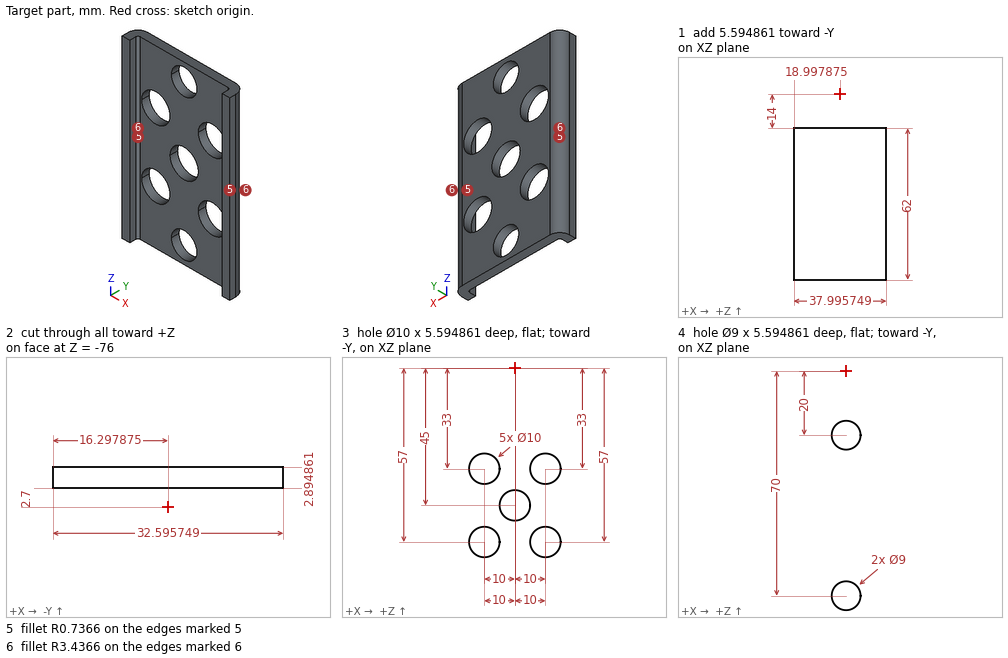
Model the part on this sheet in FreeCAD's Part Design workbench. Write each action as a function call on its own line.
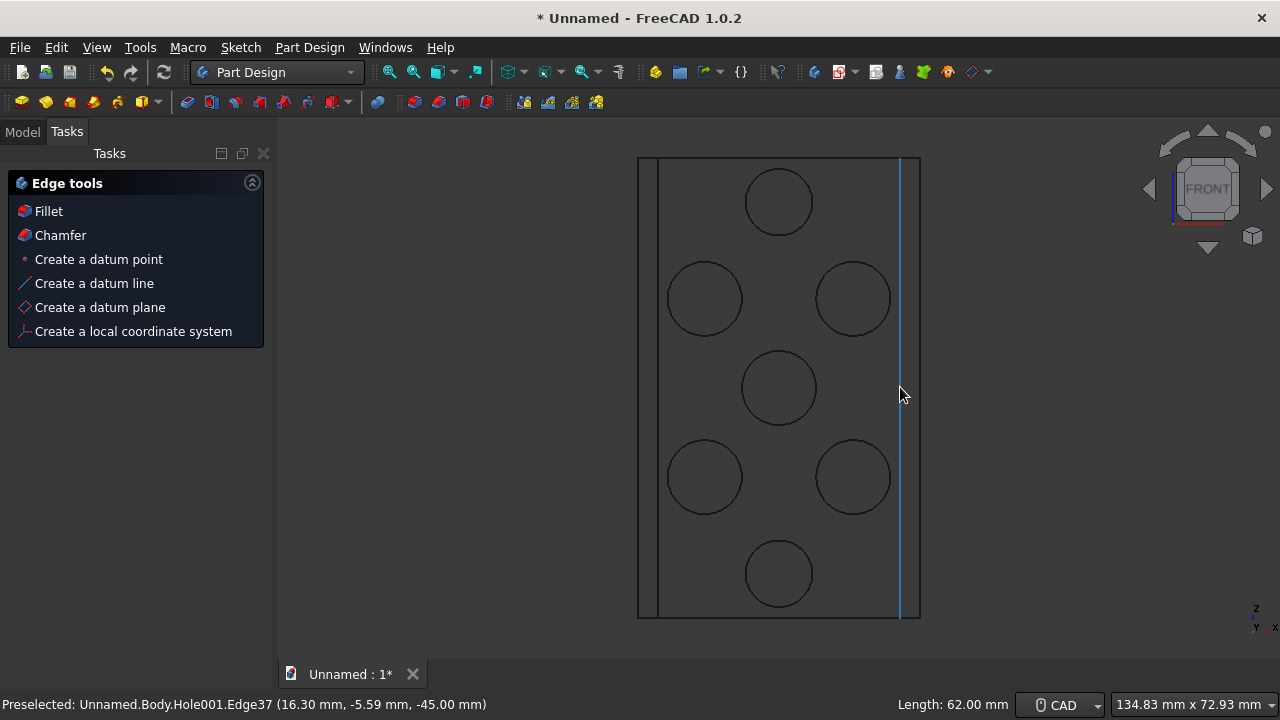
key(3)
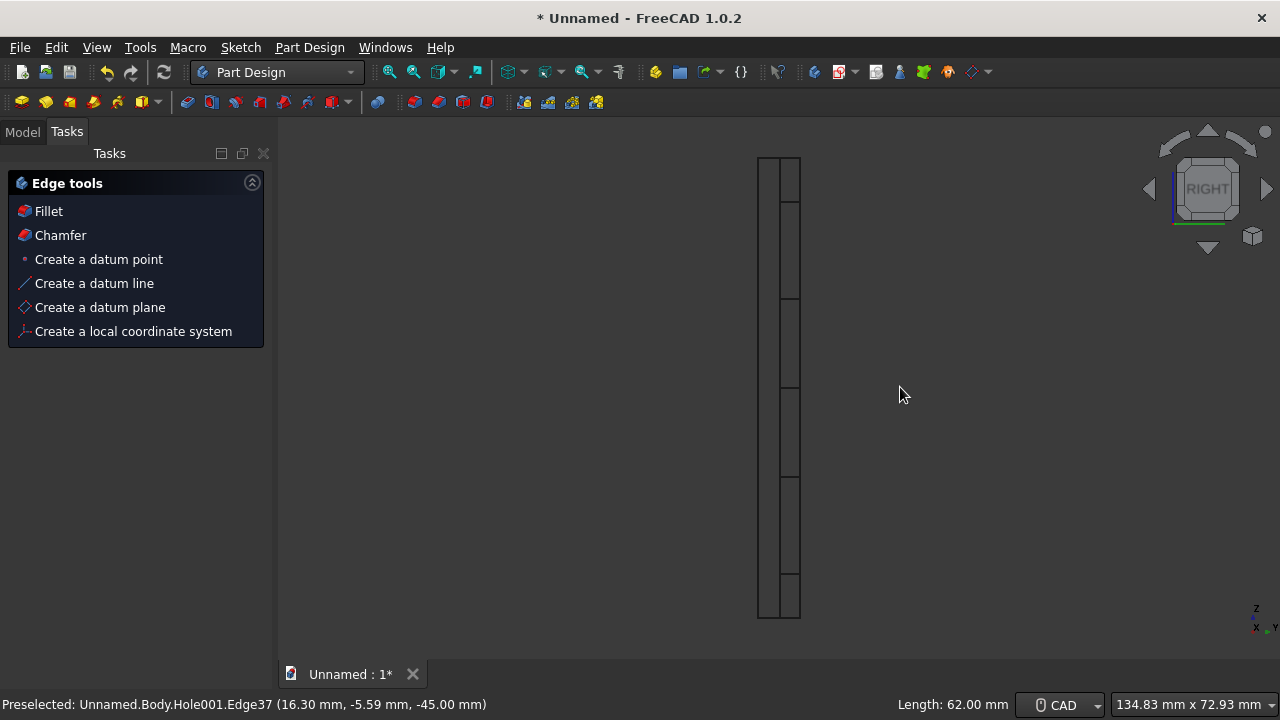
click(780, 387, ctrl)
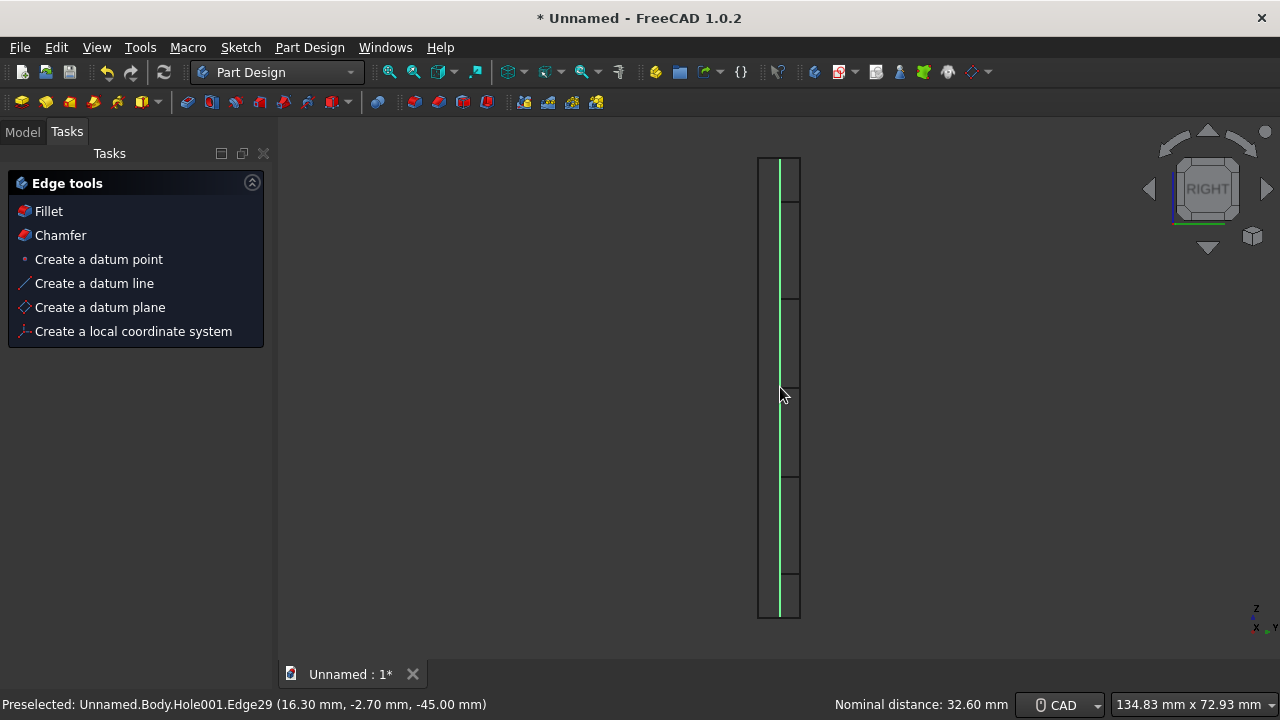
key(v)
key(1)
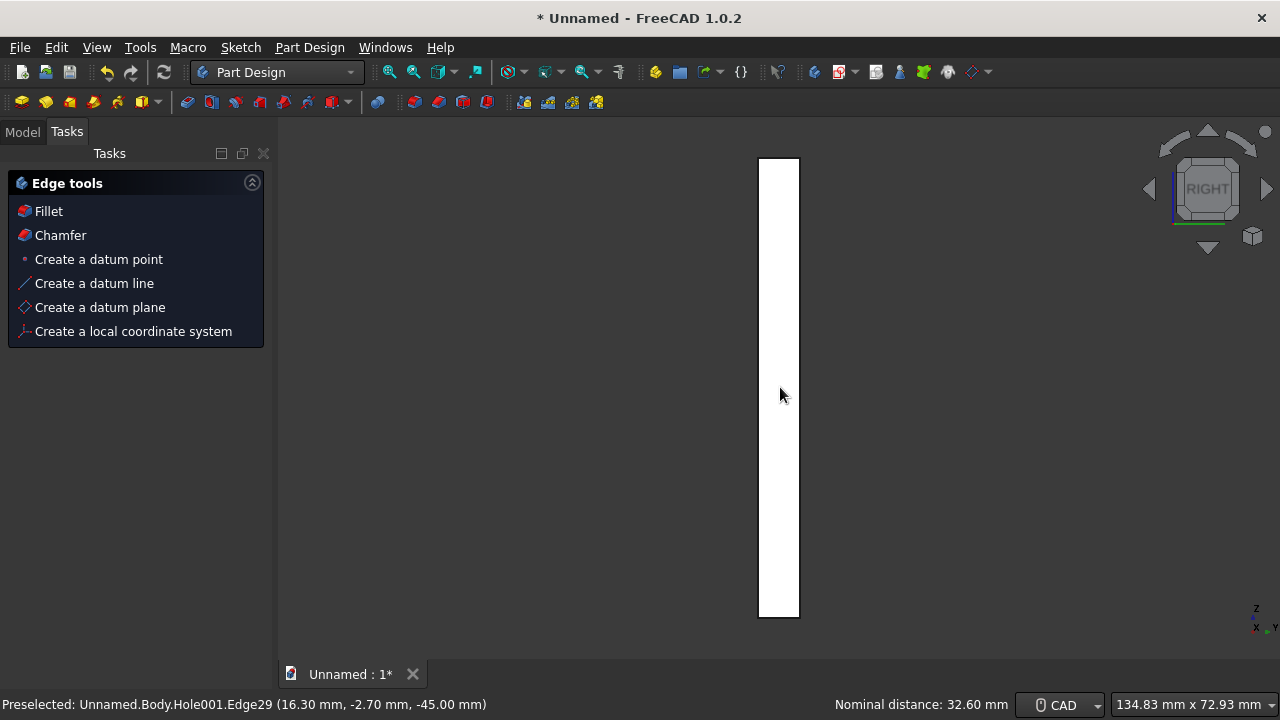
click(416, 102)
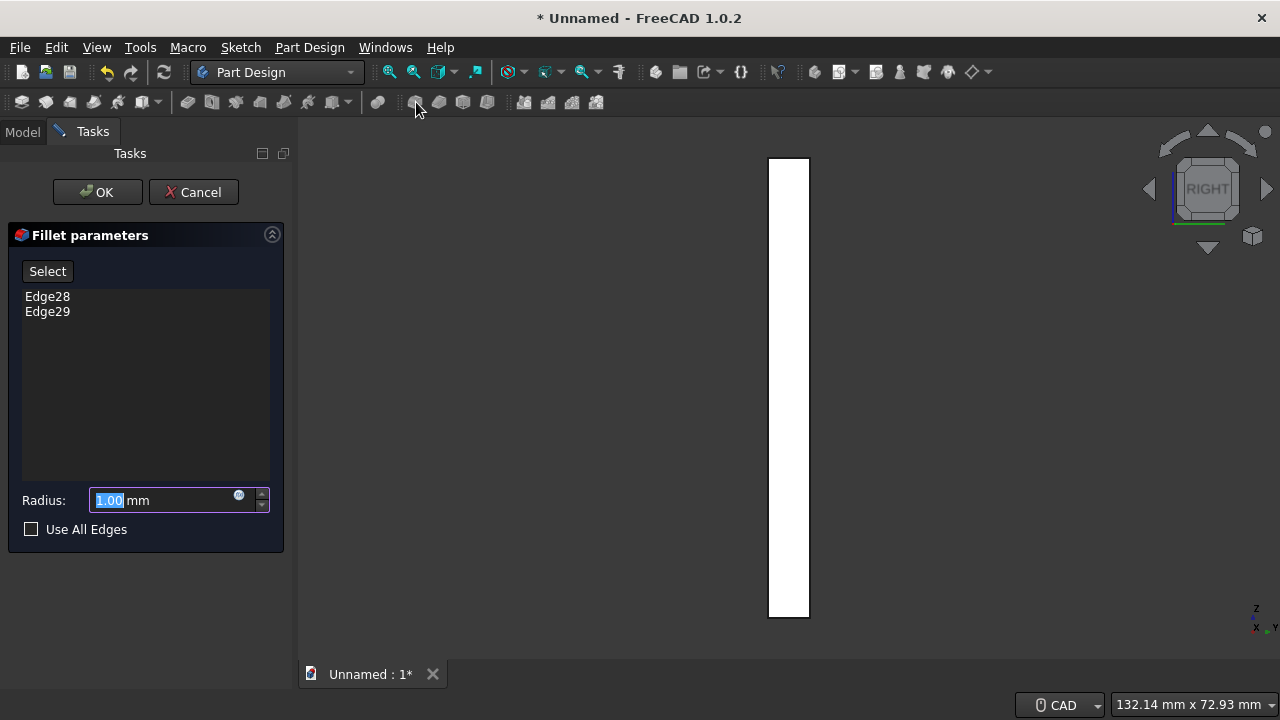
text(0.7366)
key(Tab)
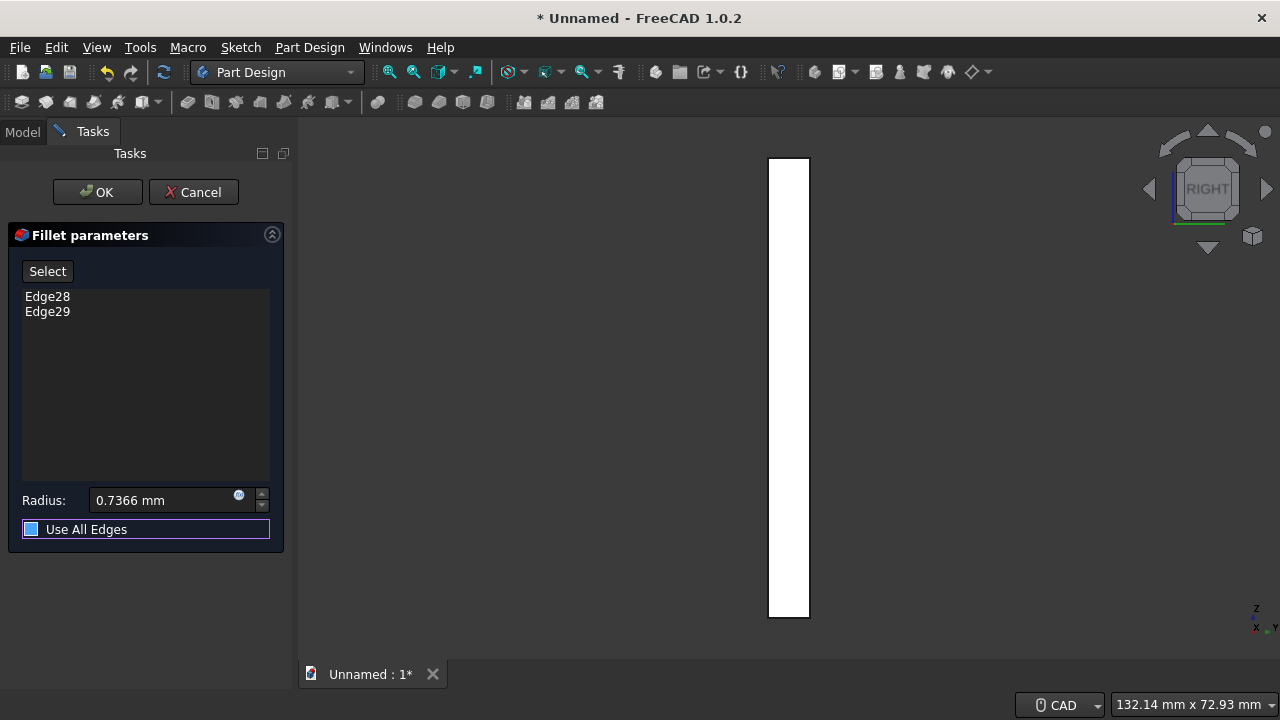
click(98, 192)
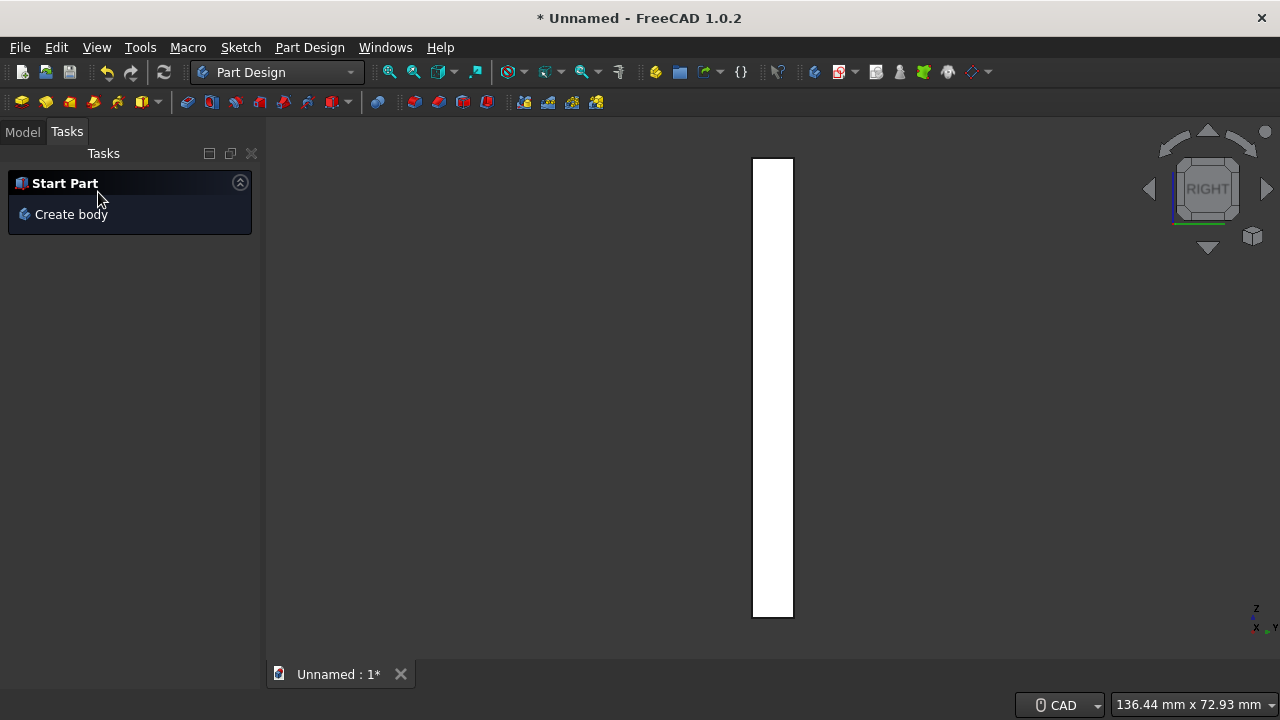
click(794, 387)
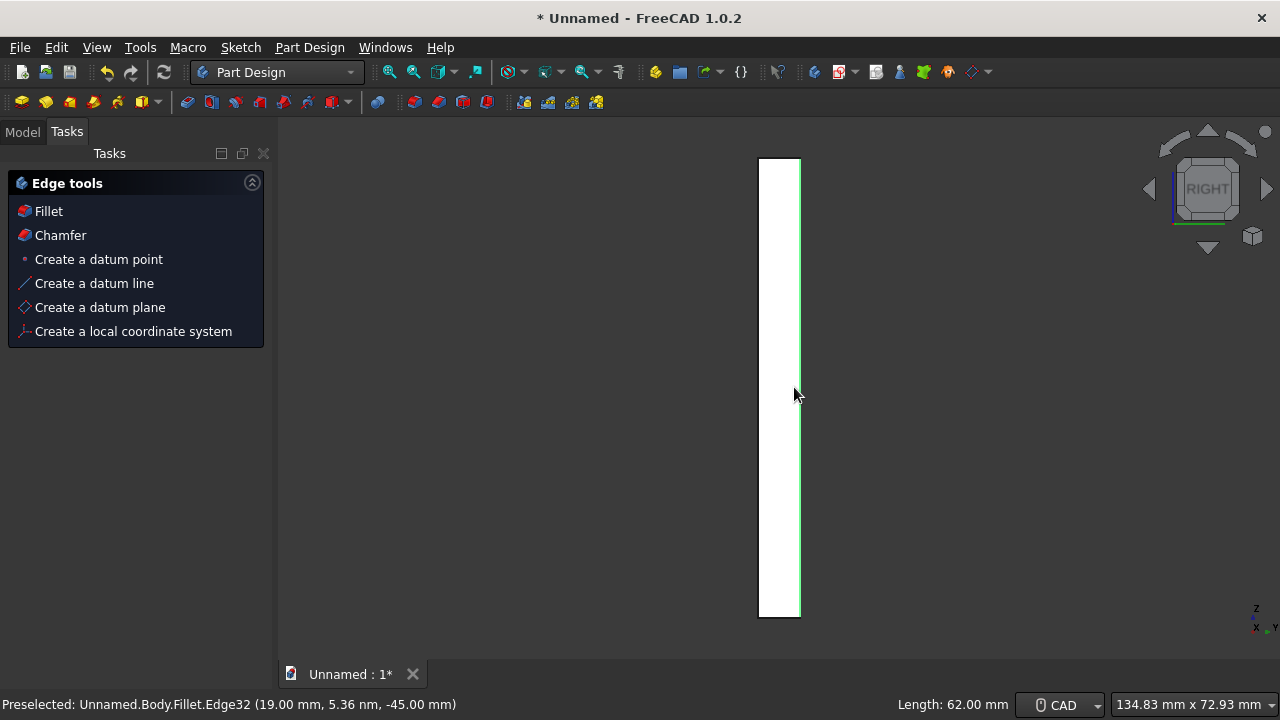
key(0)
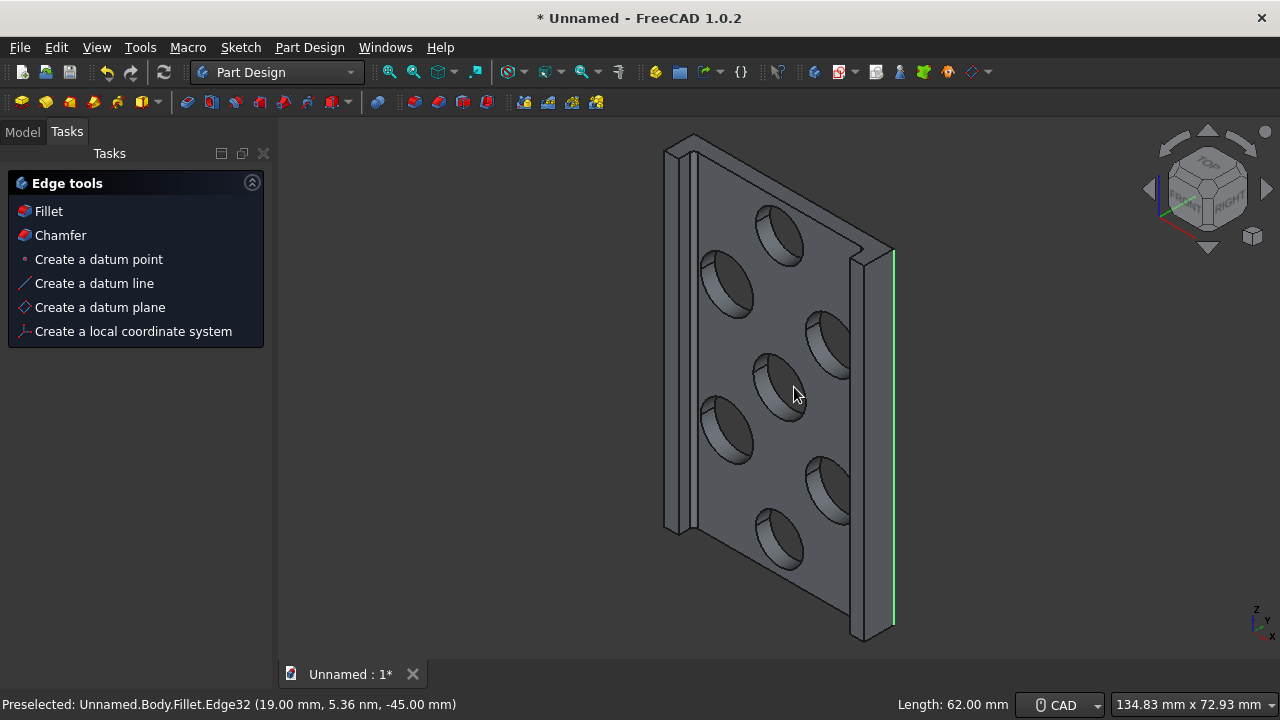
key(2)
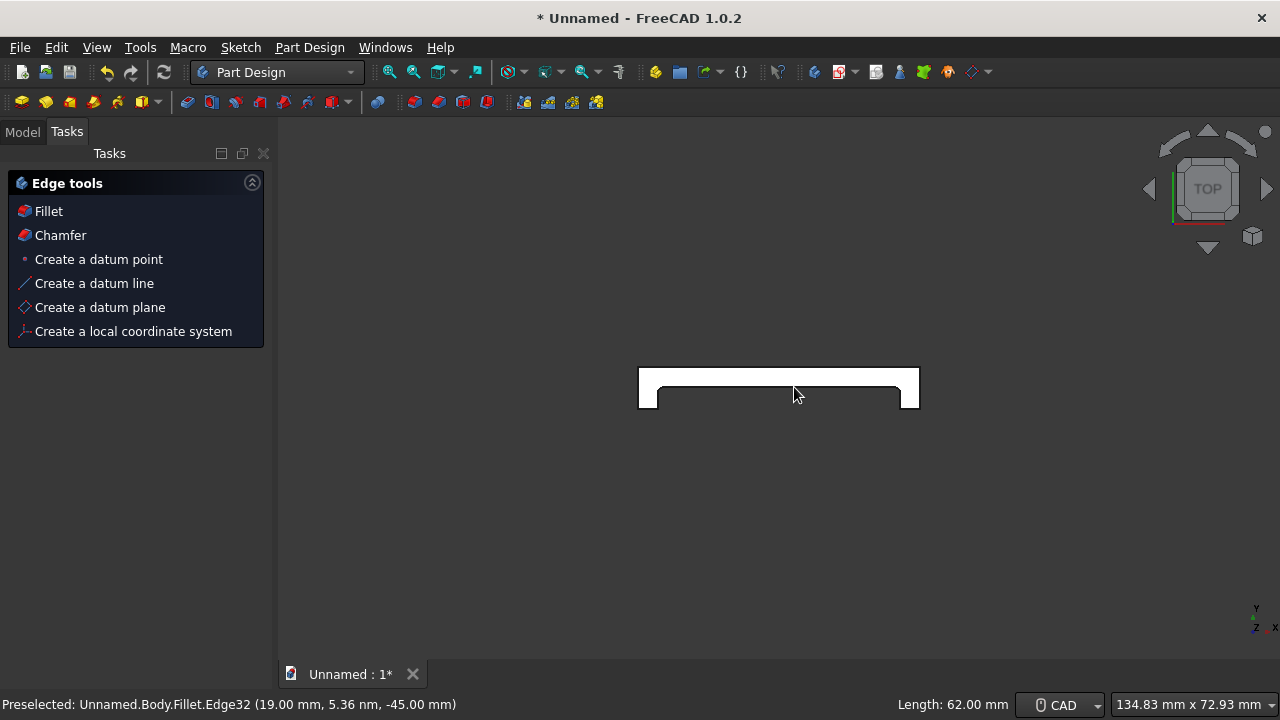
click(390, 72)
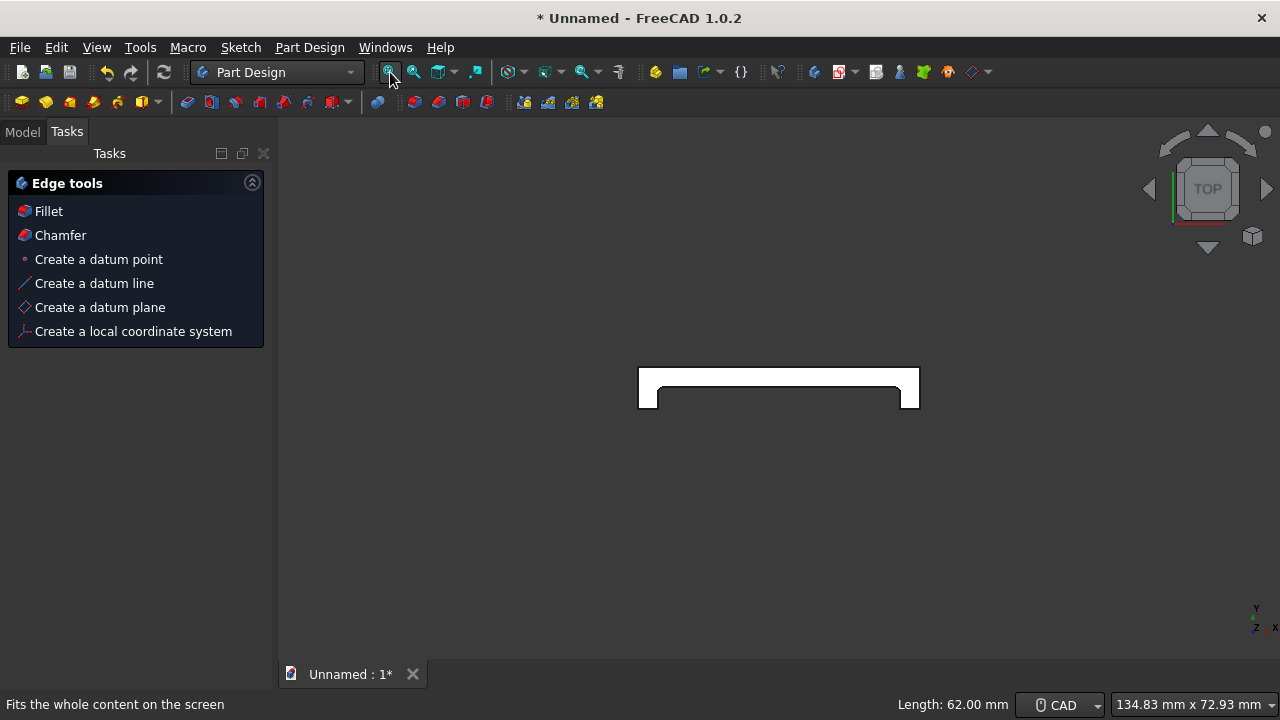
key(1)